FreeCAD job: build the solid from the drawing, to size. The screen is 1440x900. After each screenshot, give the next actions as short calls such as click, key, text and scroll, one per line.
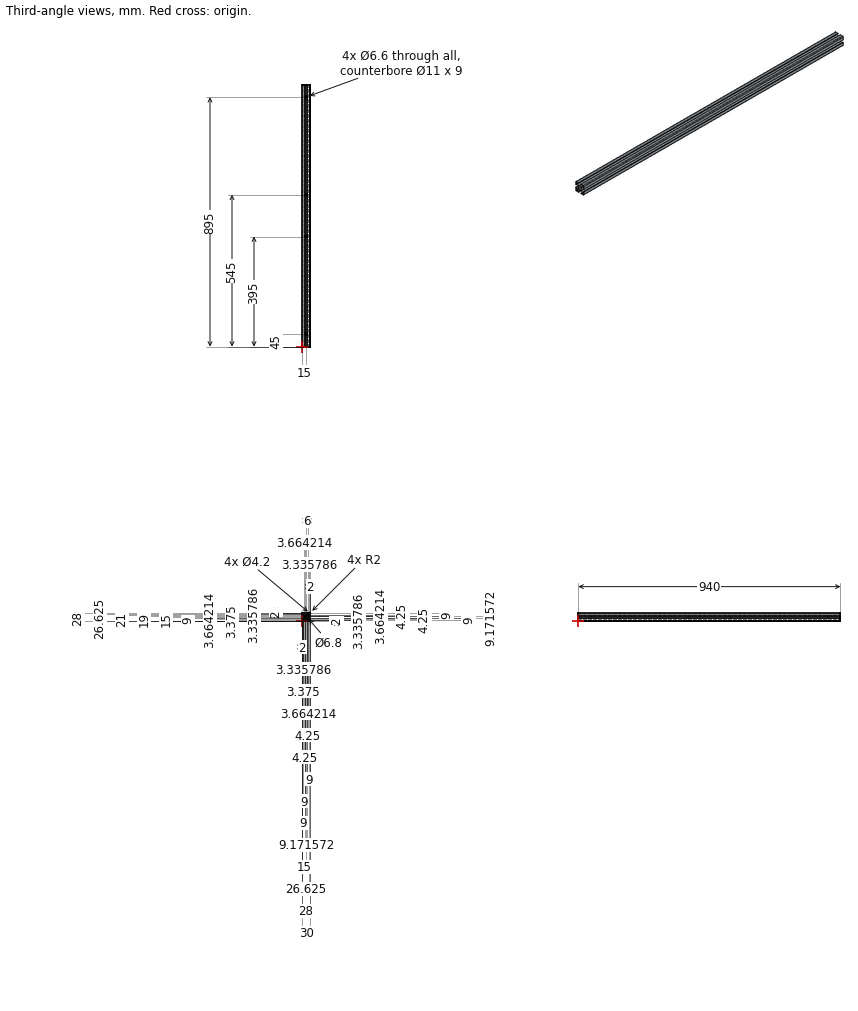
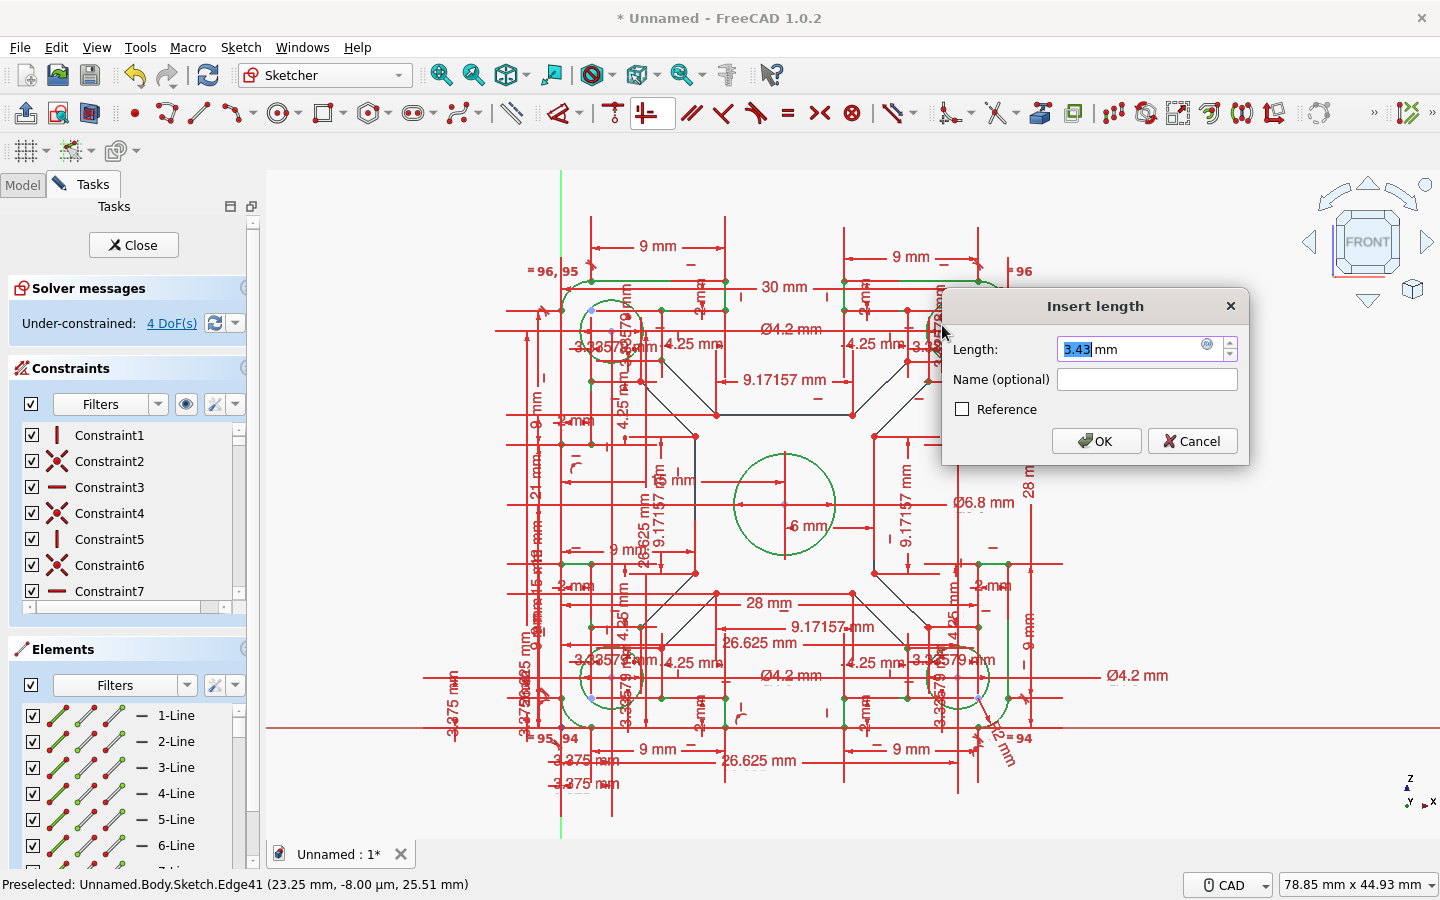
text(3.335786)
key(Return)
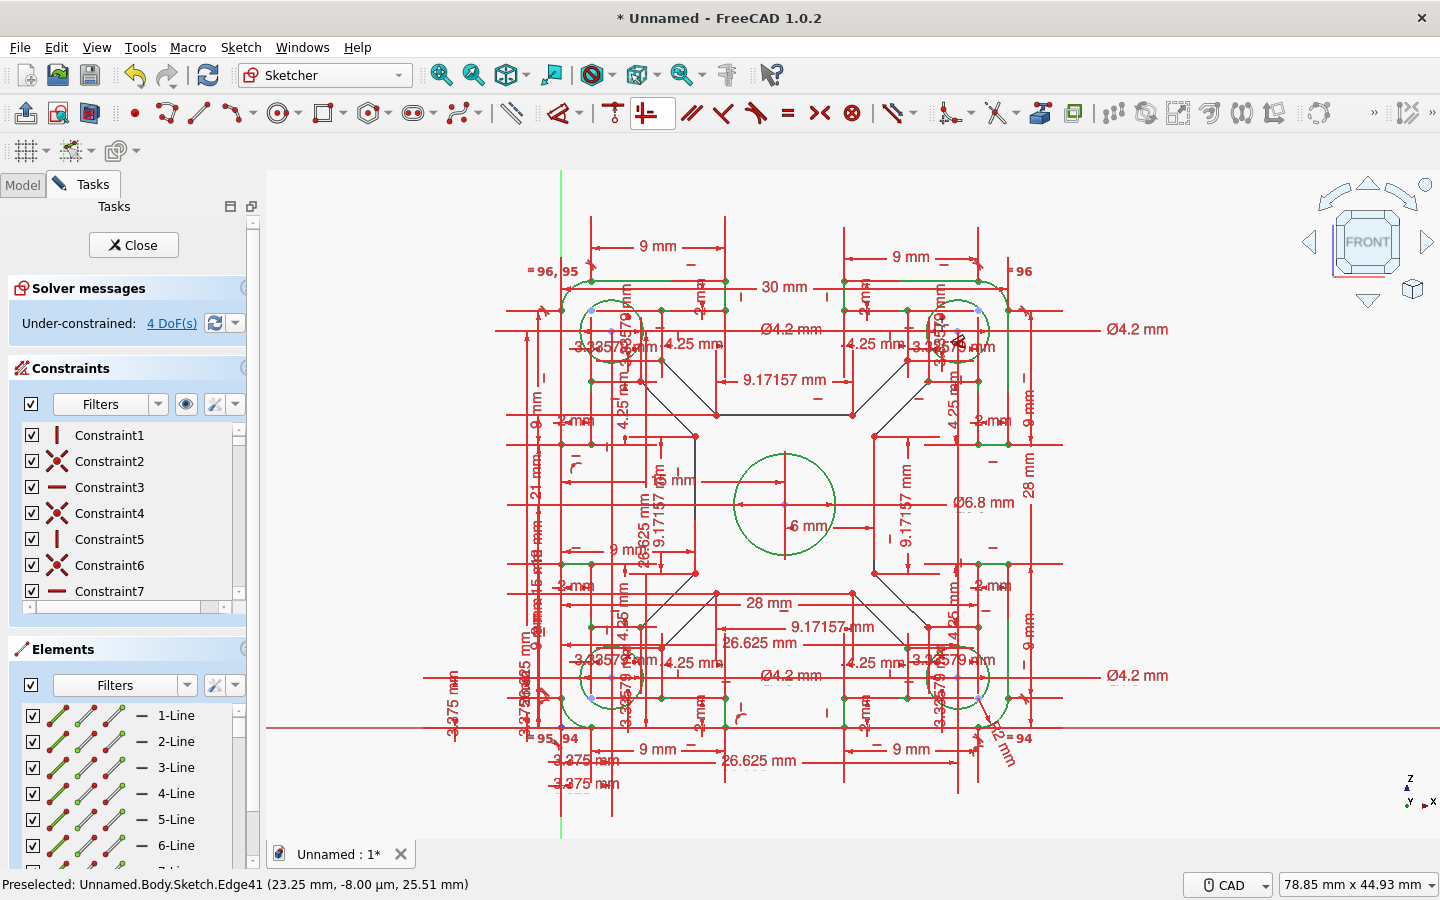
click(912, 398)
click(840, 429)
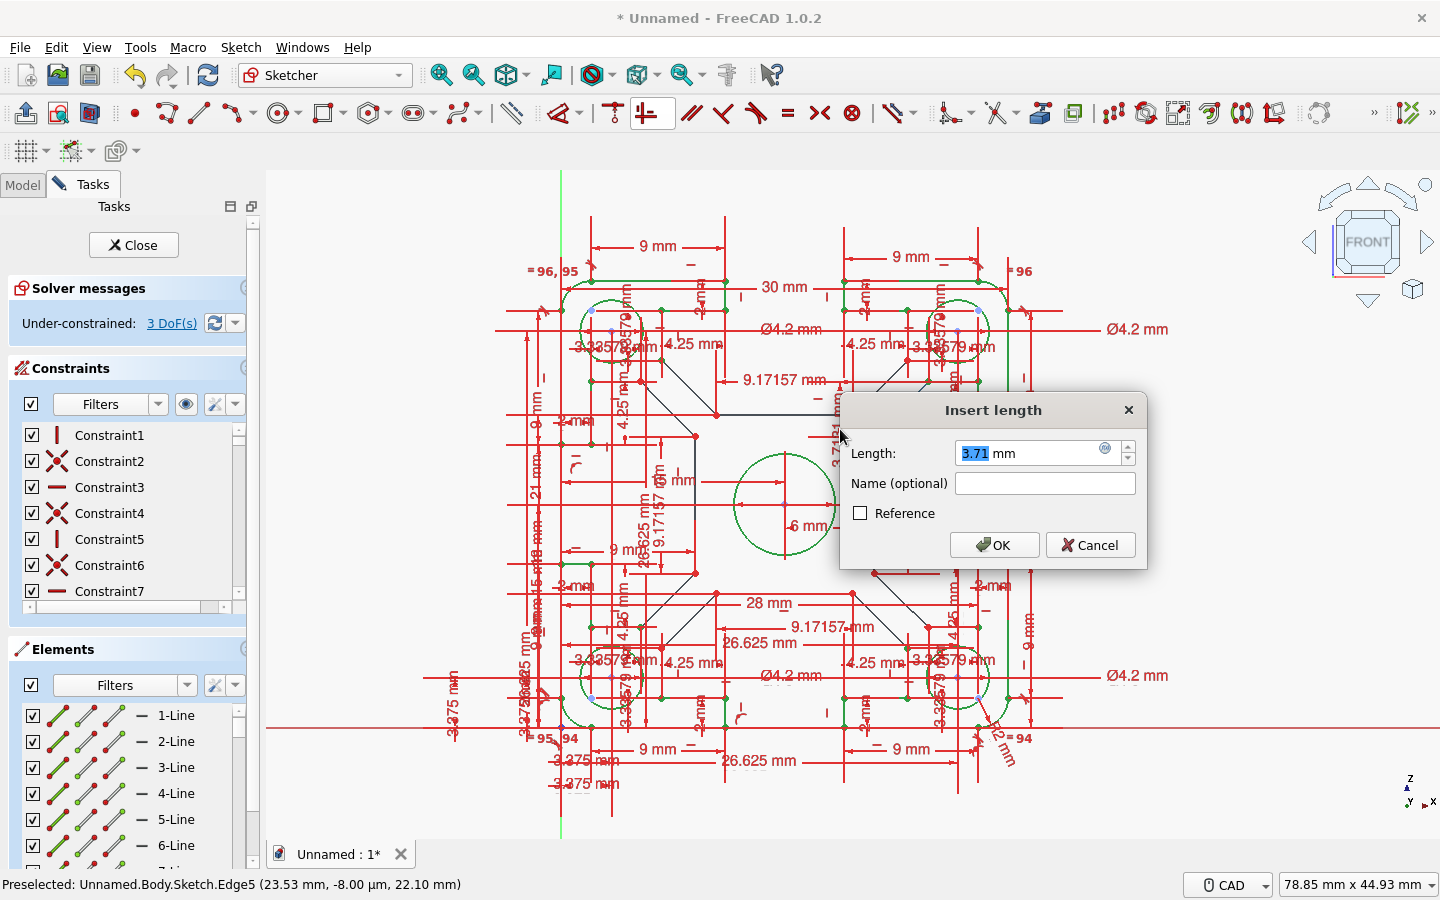
text(3.664214)
key(Return)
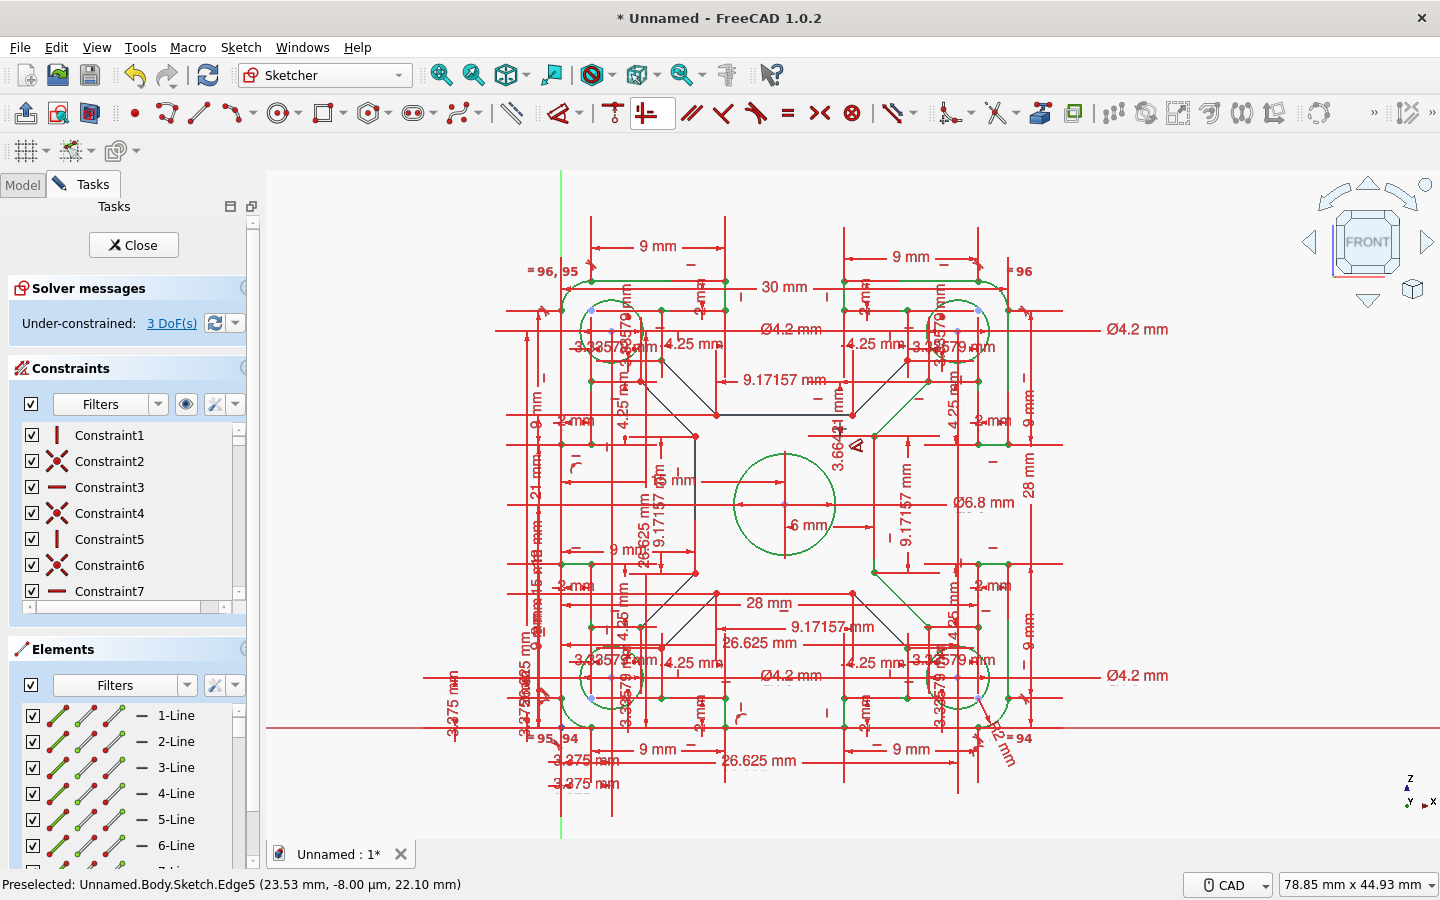
click(891, 632)
click(893, 560)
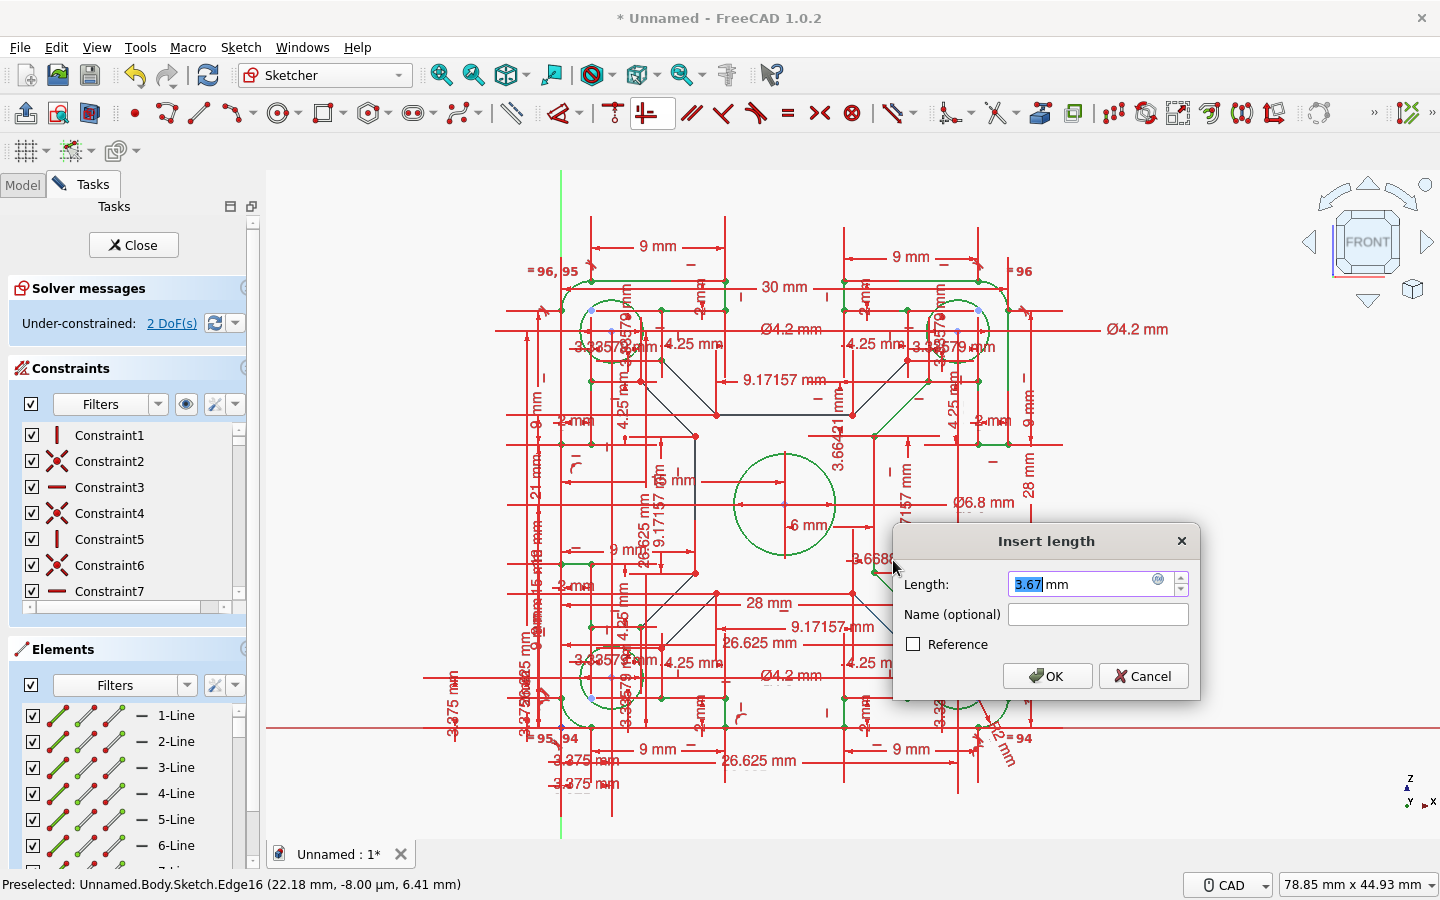
text(3.664214)
key(Return)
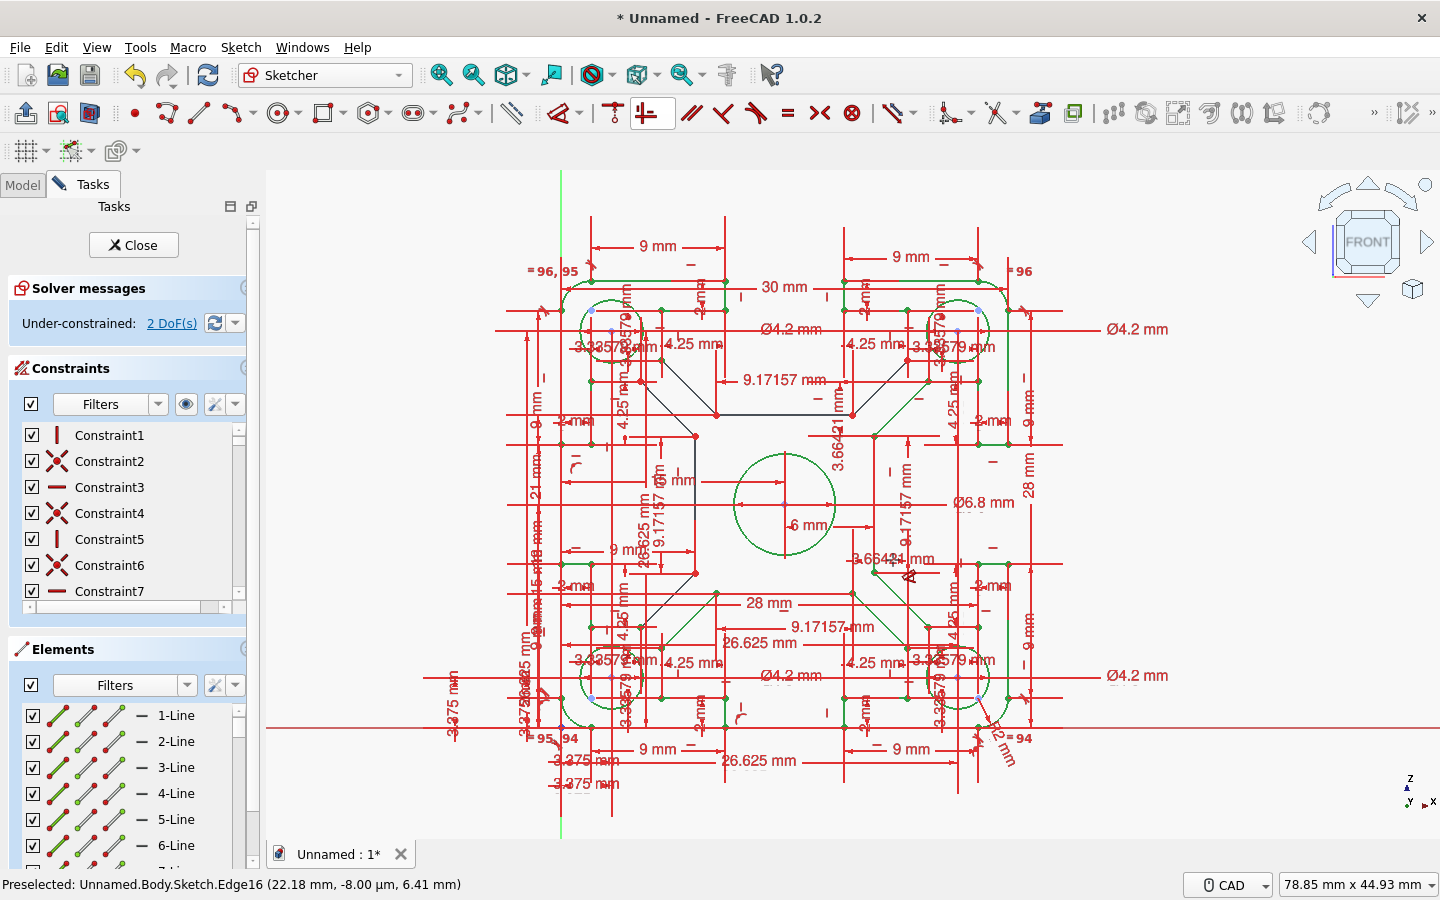
click(657, 611)
click(461, 600)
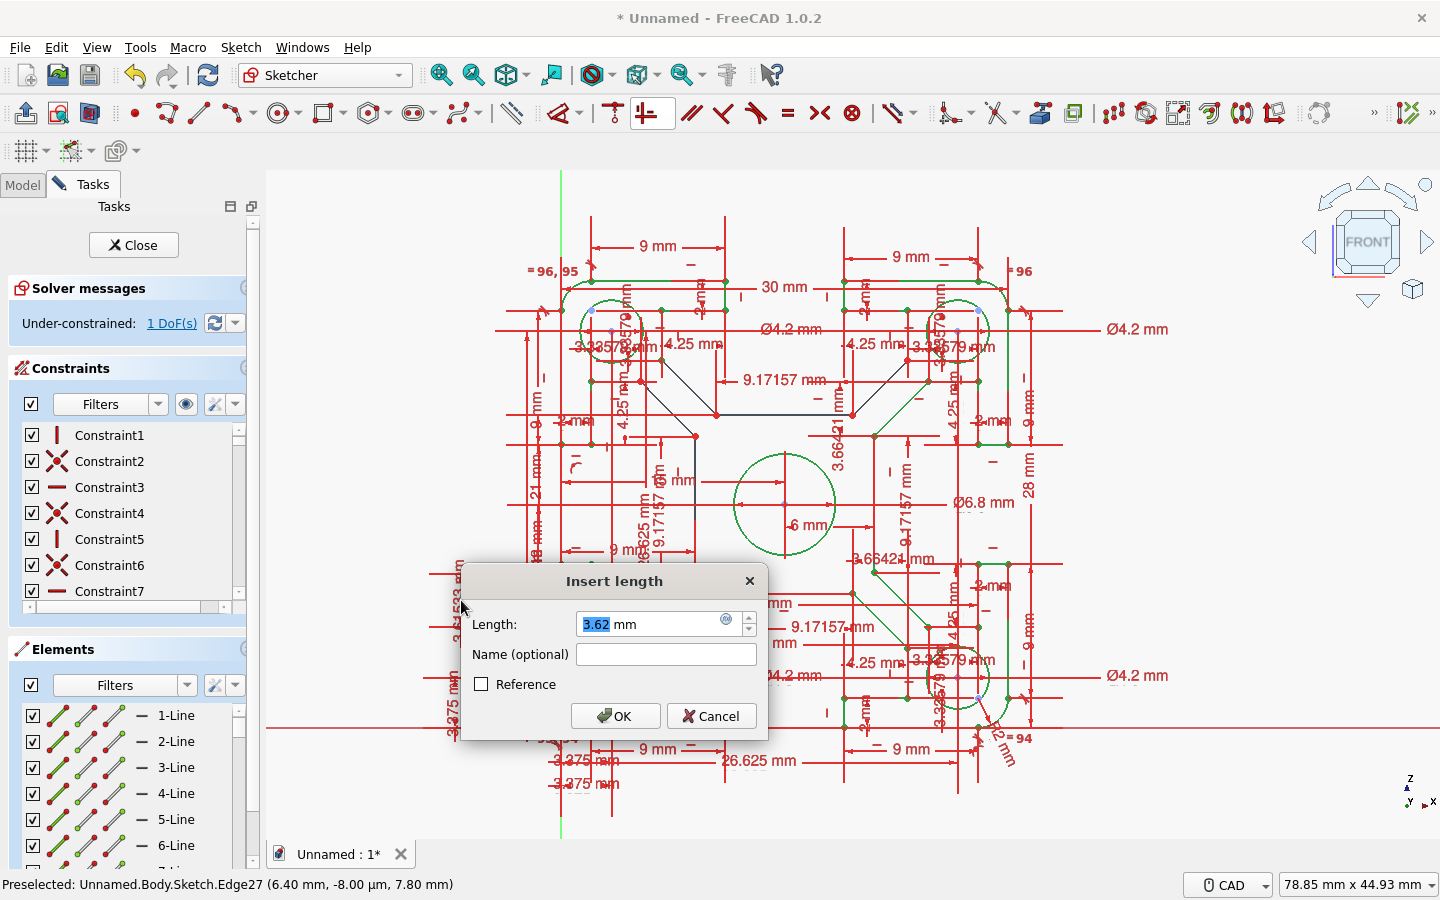
text(3.664214)
key(Return)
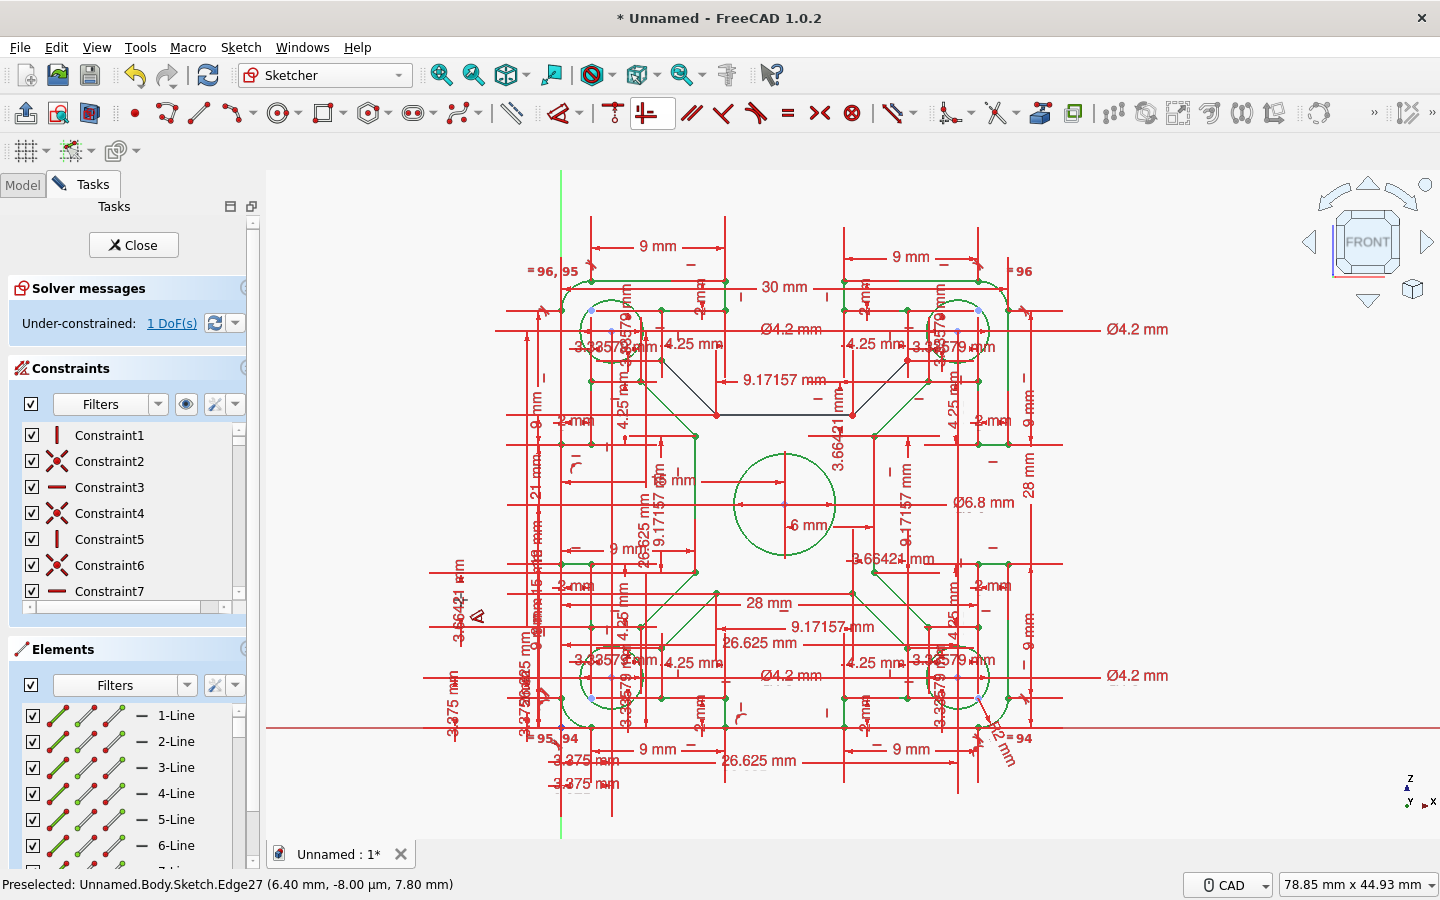
click(678, 377)
click(677, 449)